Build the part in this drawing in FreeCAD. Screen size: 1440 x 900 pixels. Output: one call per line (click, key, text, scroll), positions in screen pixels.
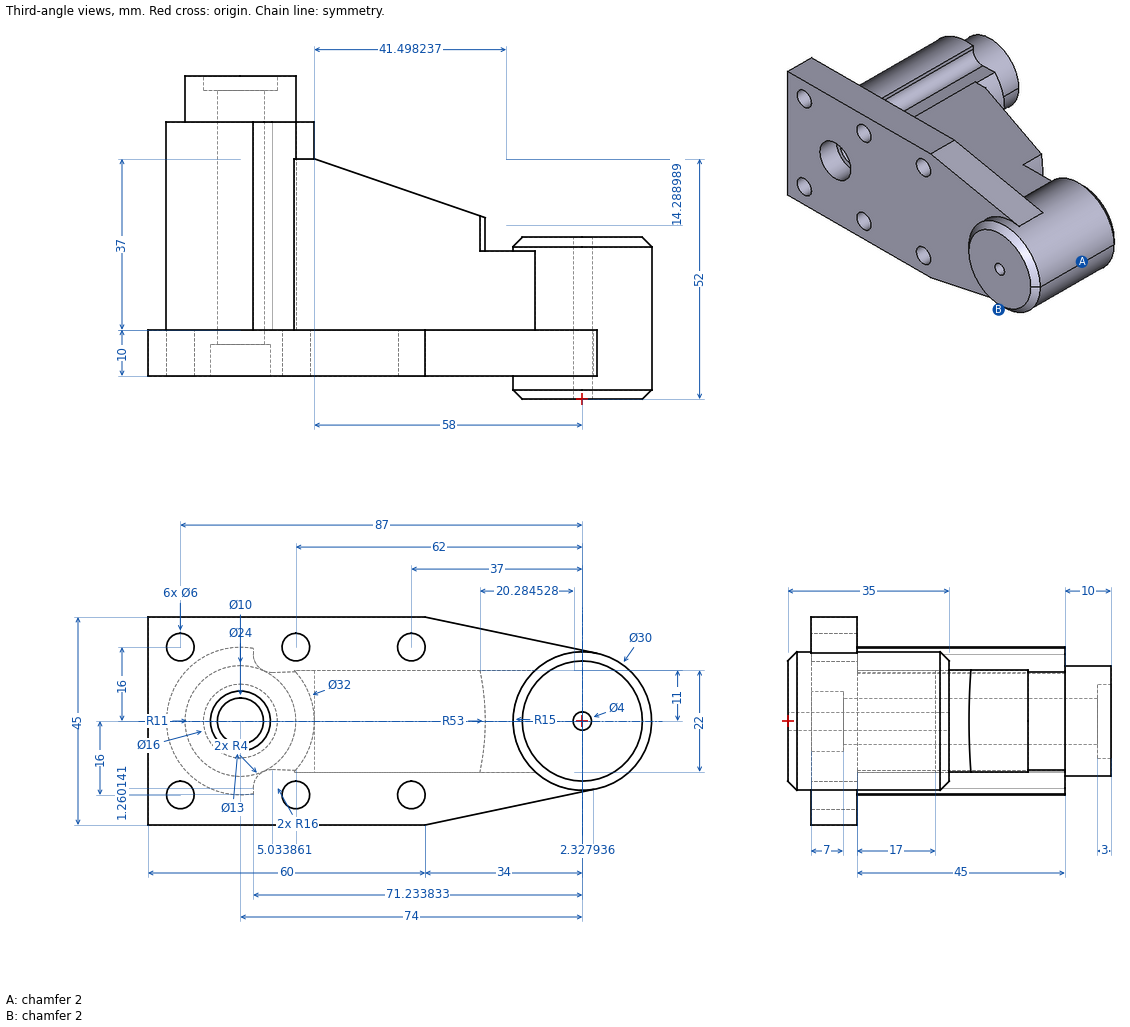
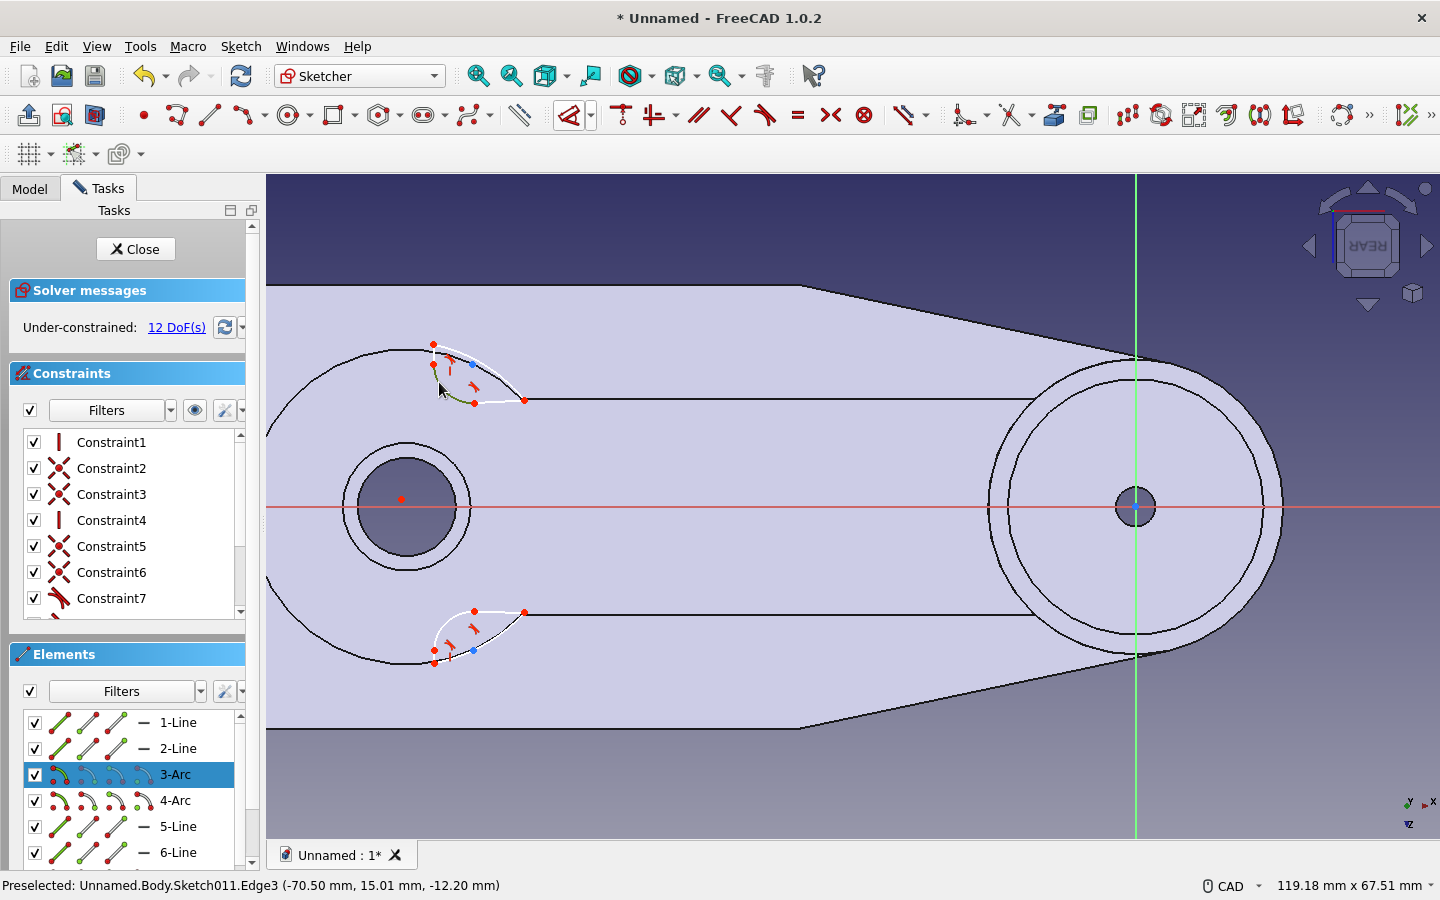
click(456, 616)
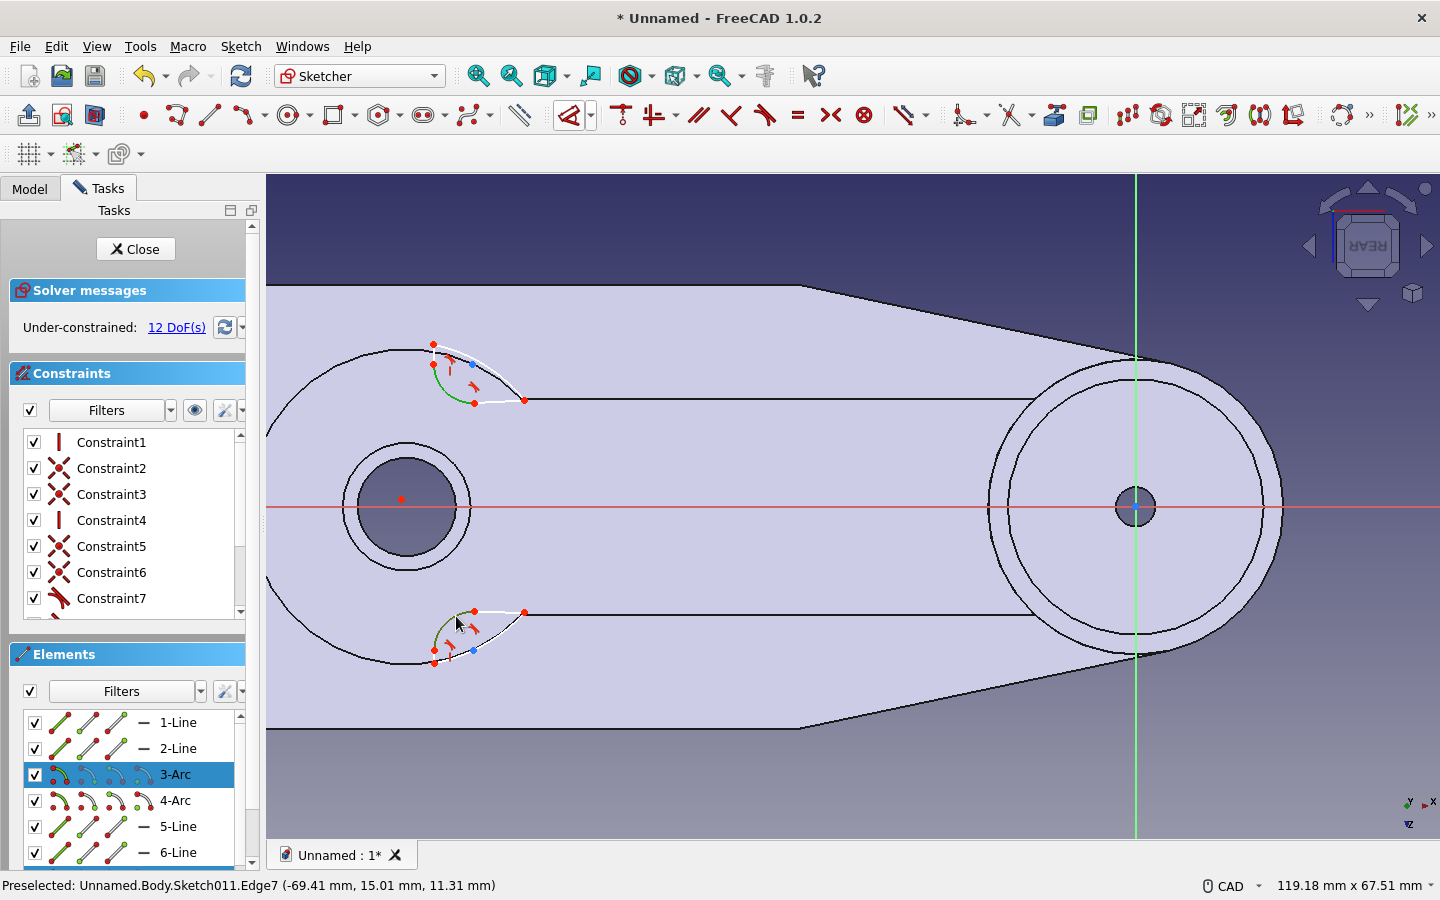
click(798, 116)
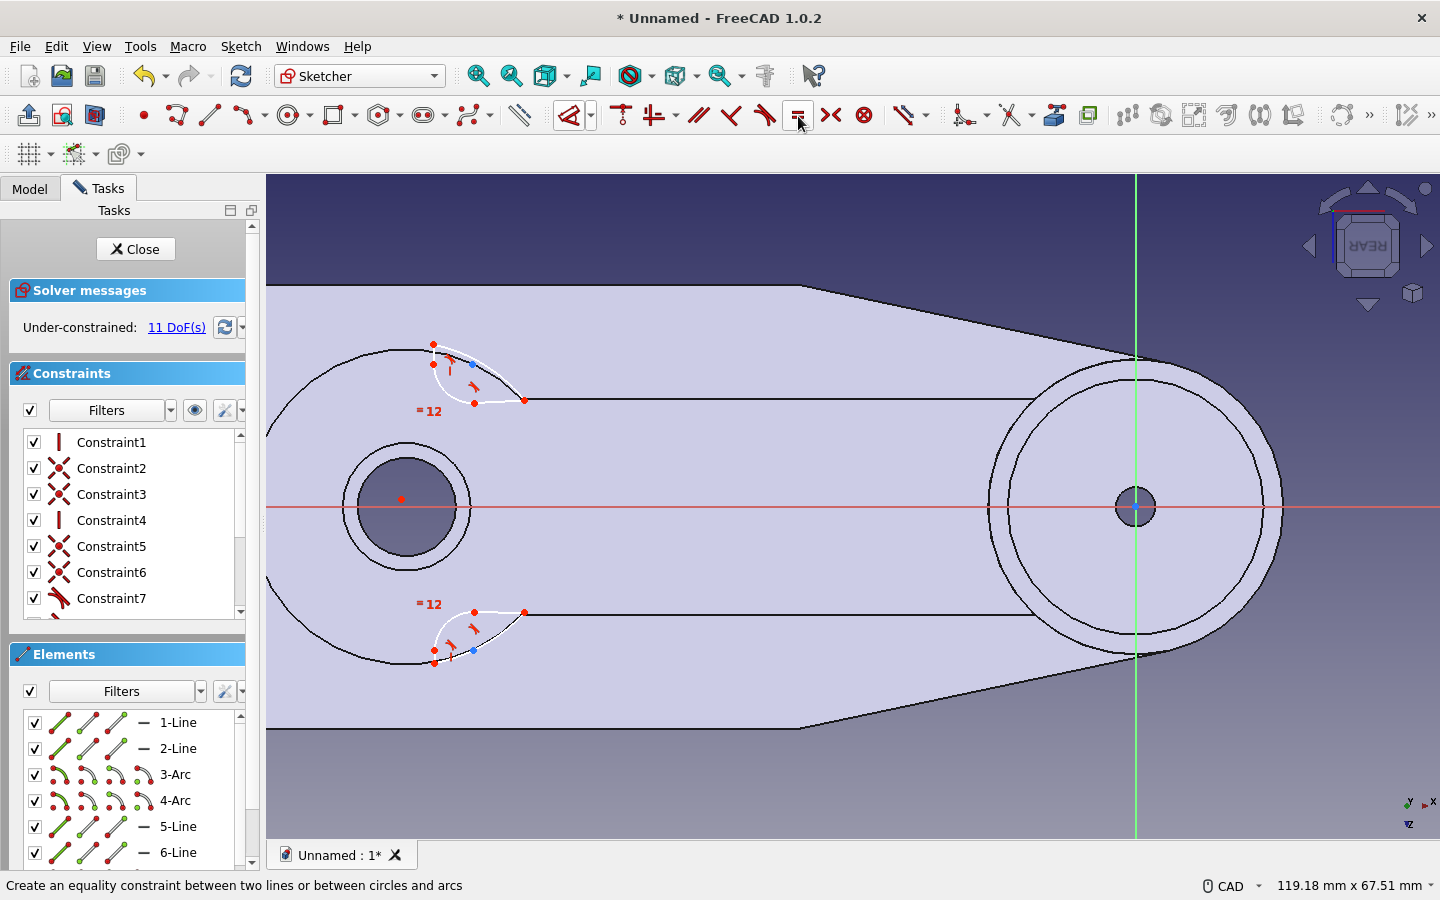
click(502, 377)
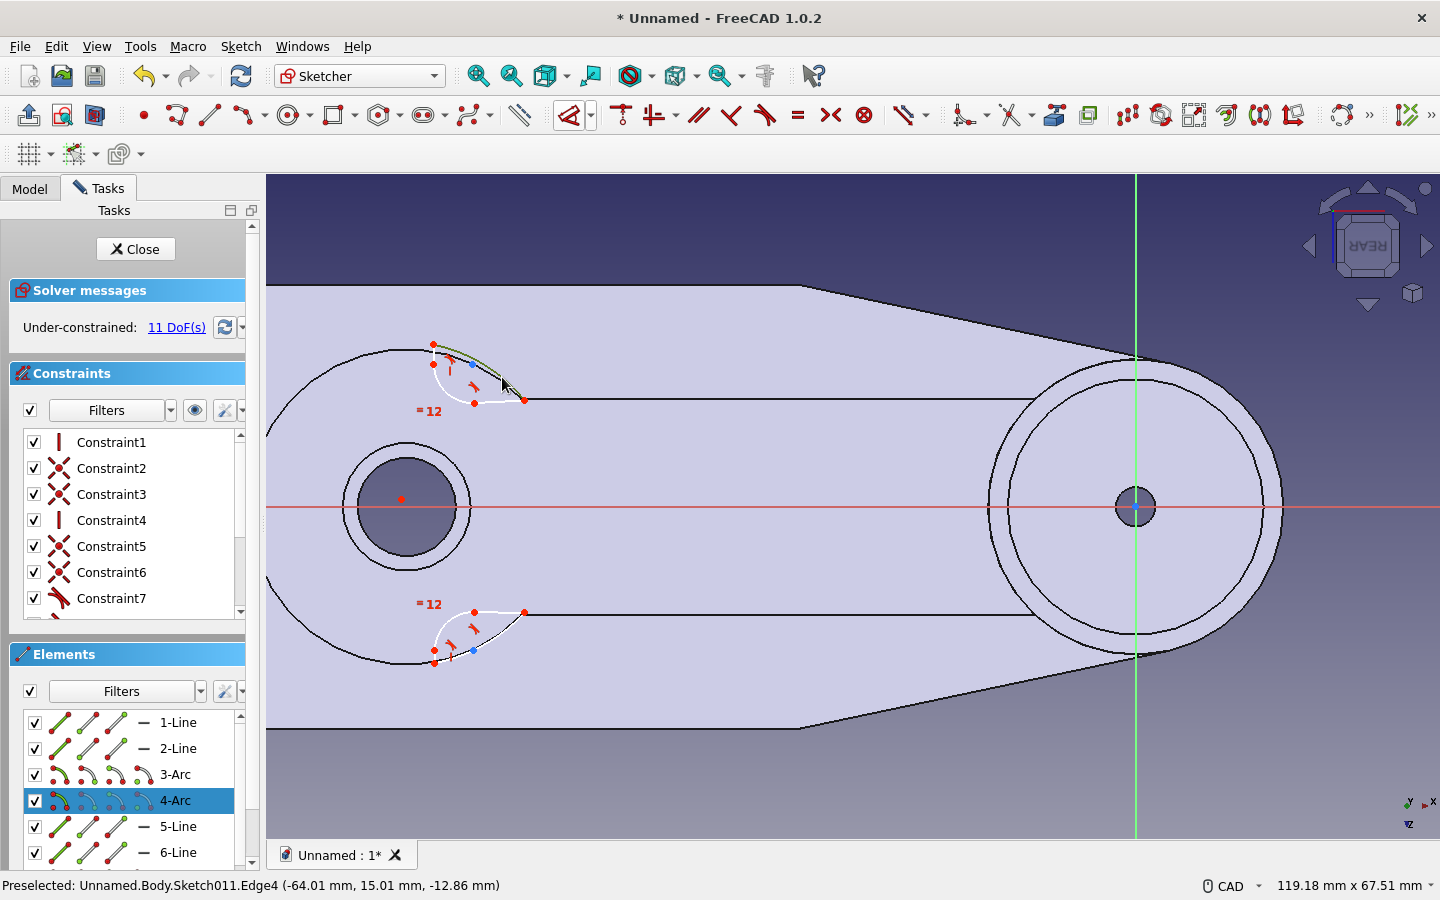
click(465, 654)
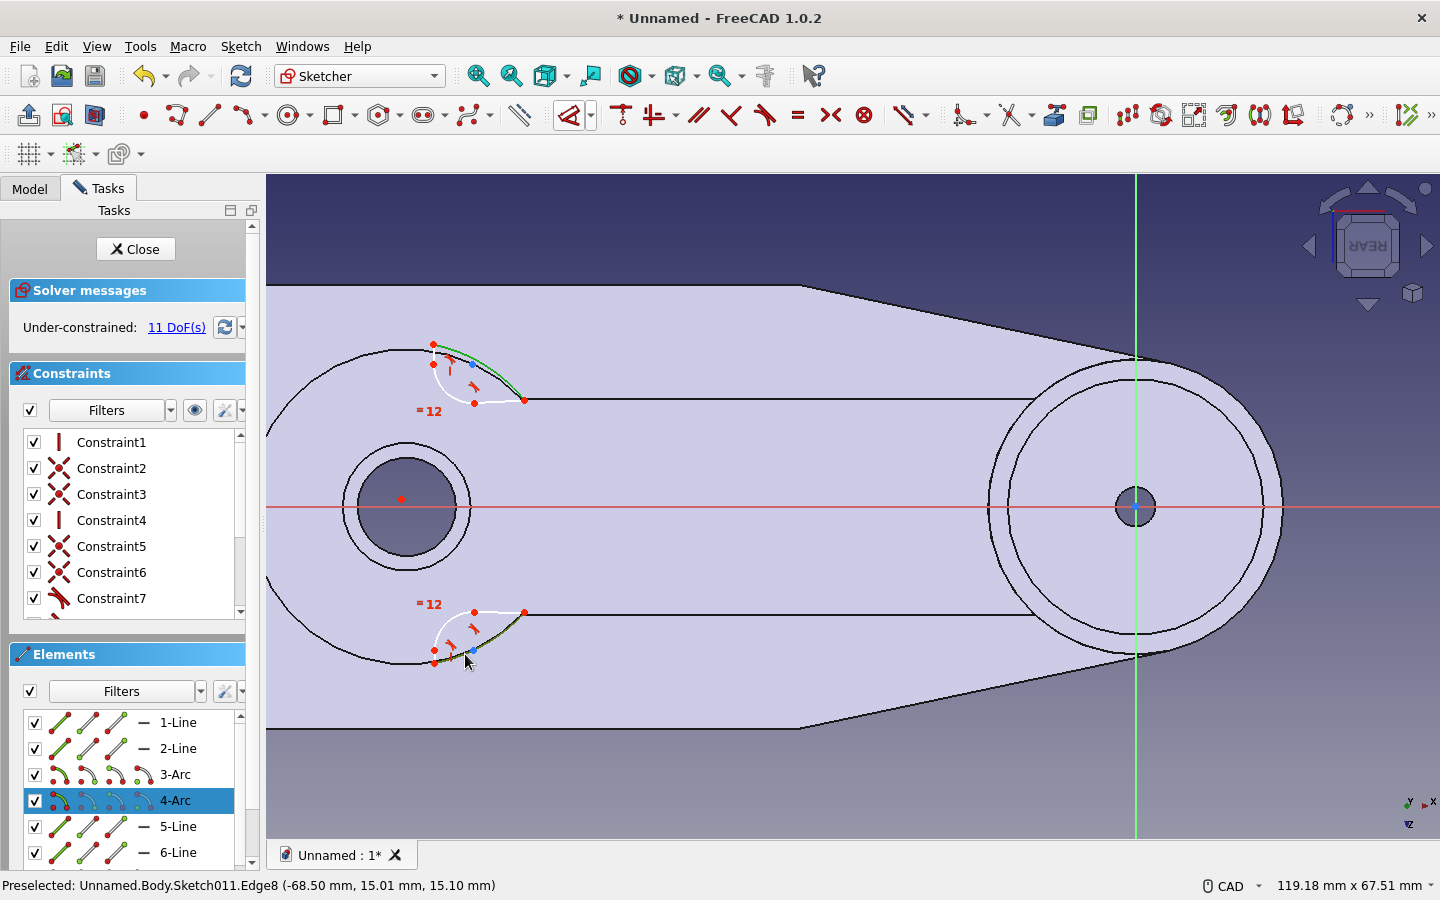
click(798, 116)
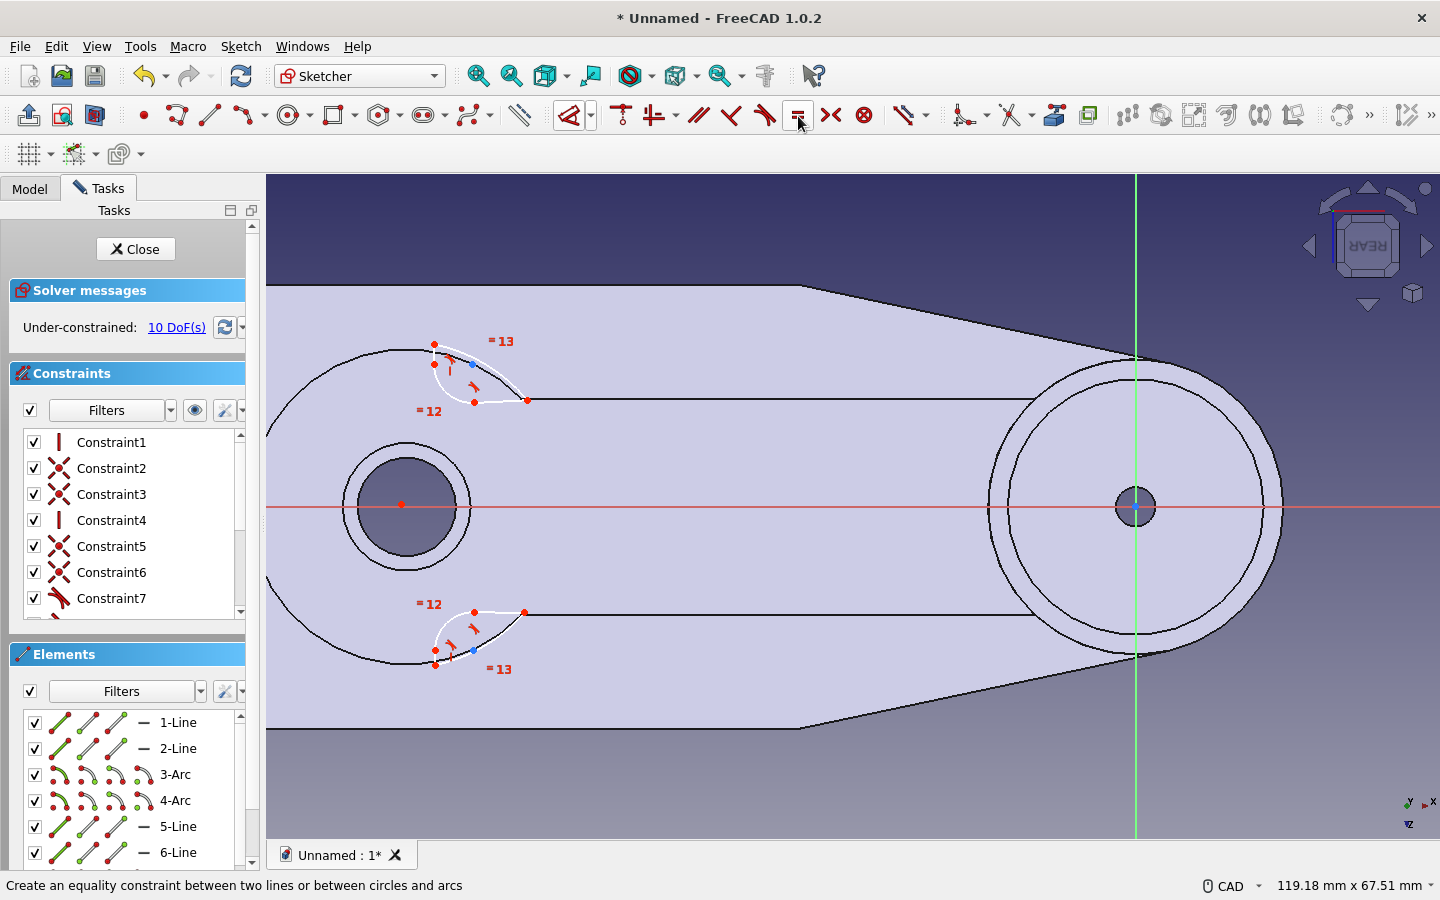
click(401, 505)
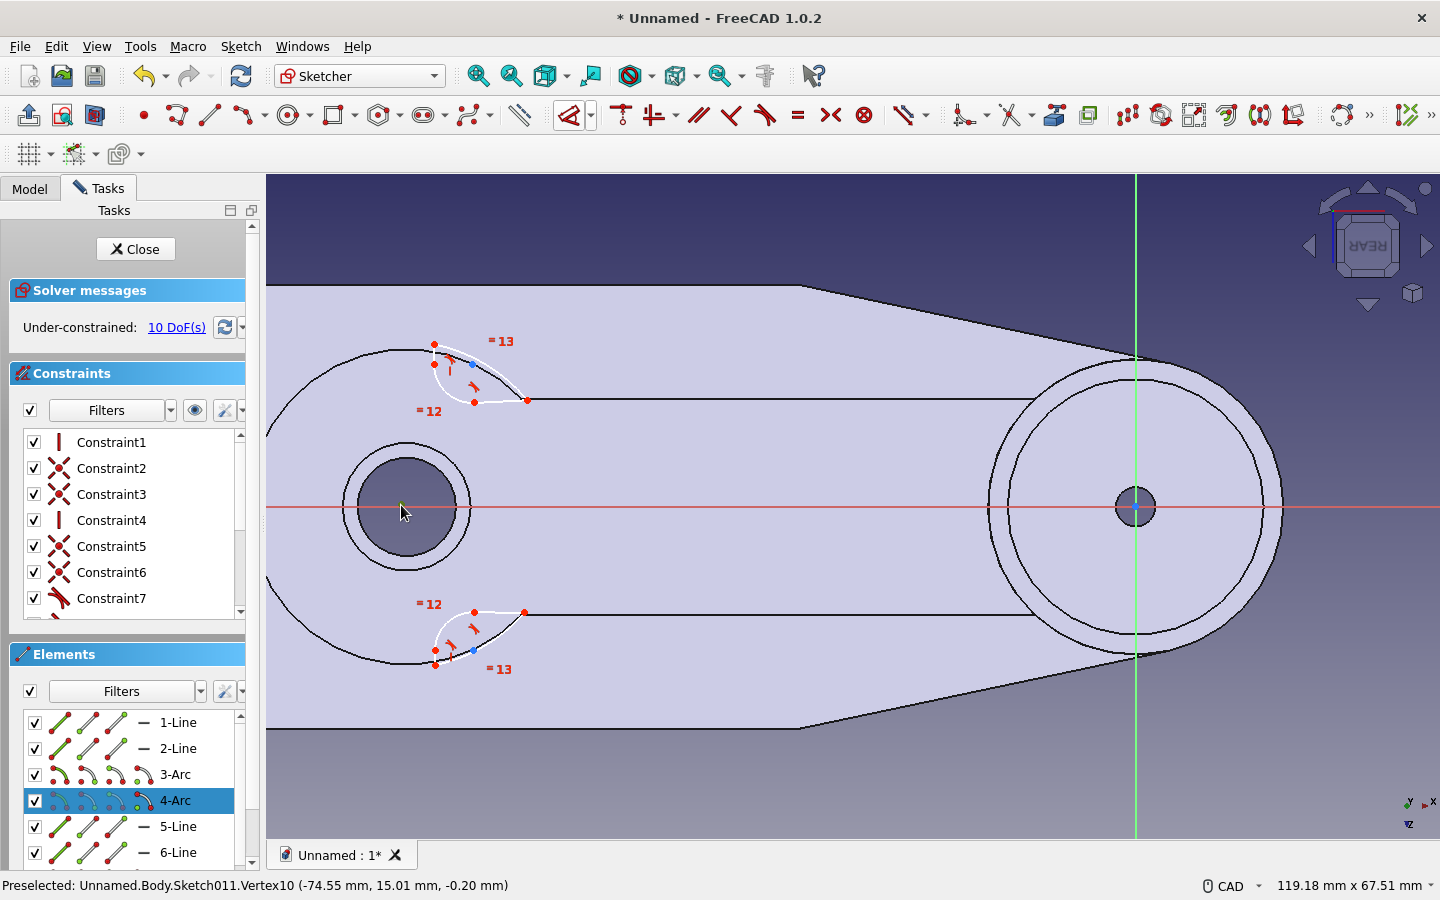
click(364, 507)